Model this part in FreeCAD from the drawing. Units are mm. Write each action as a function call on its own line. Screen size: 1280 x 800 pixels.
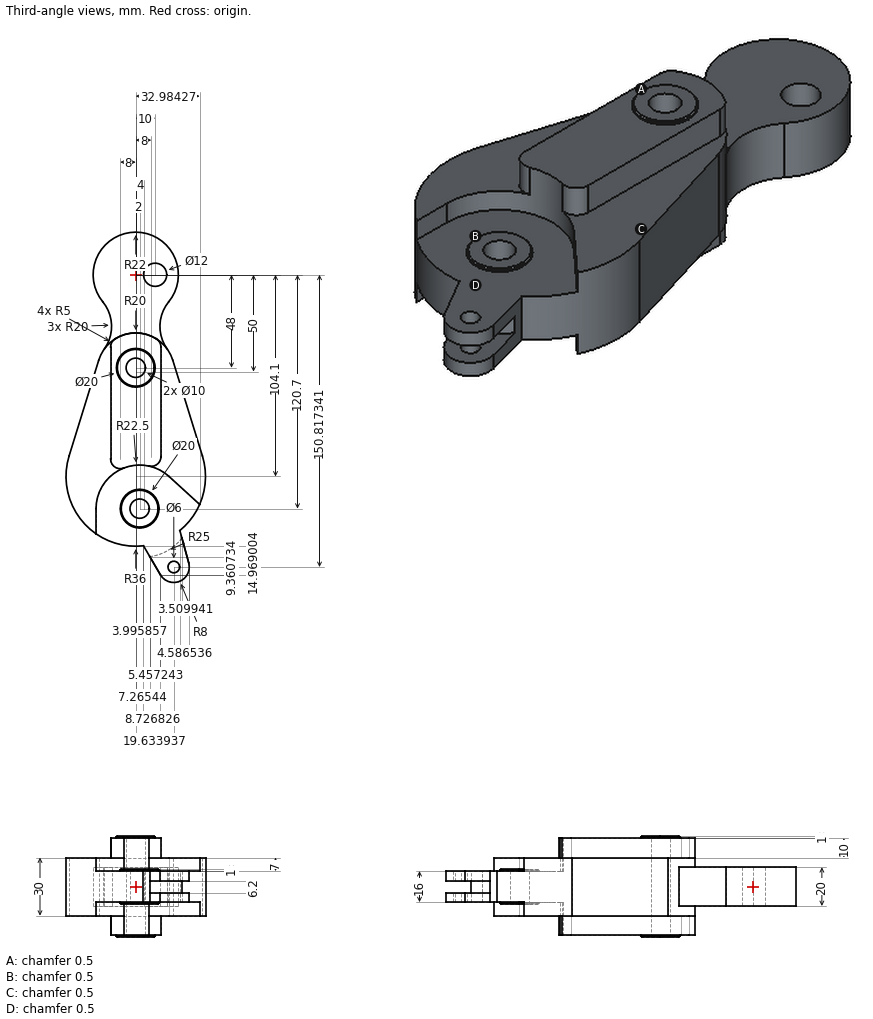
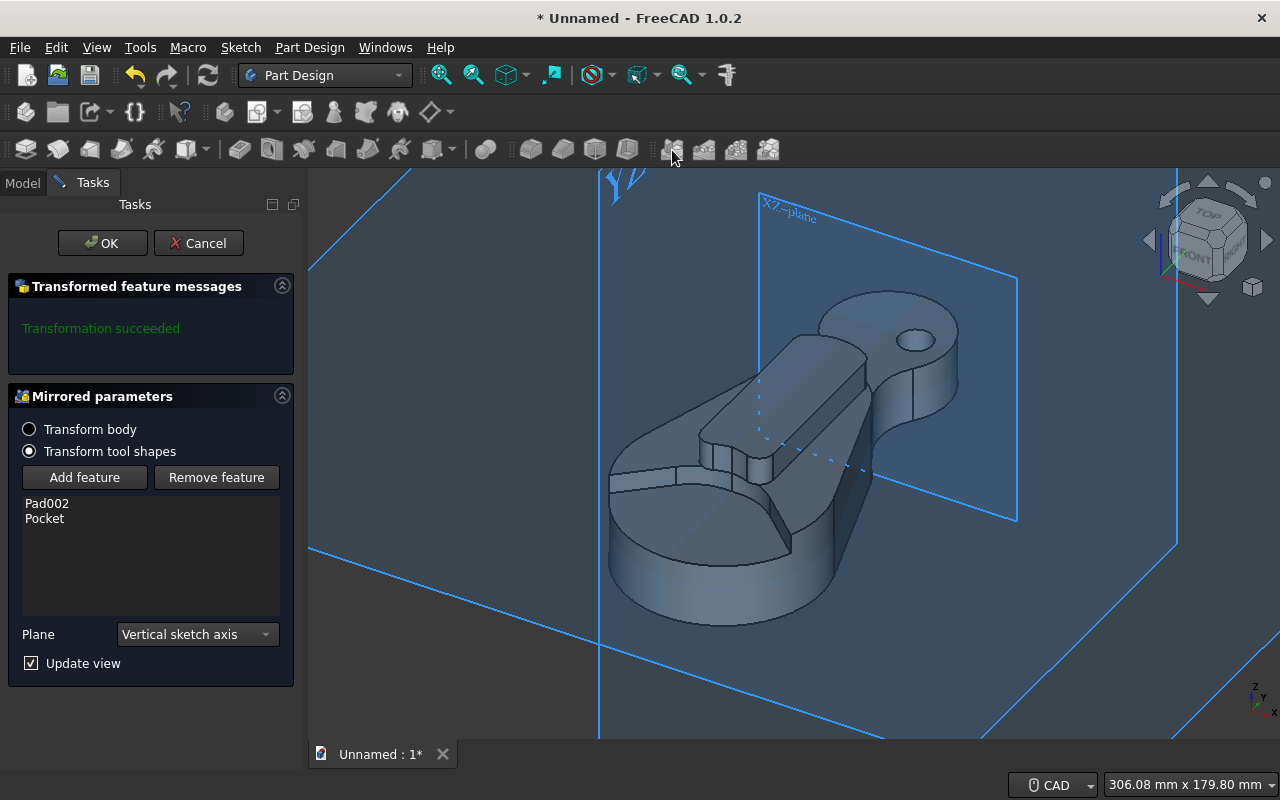
click(198, 634)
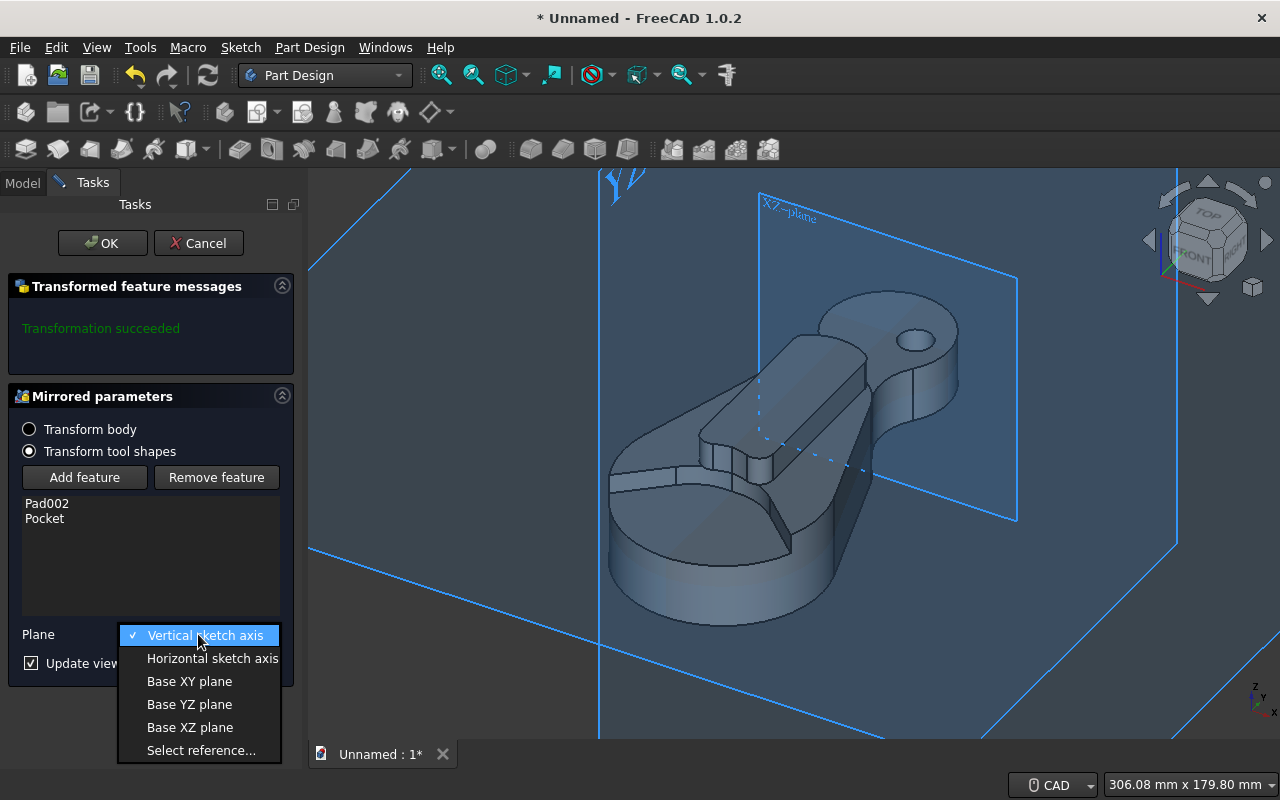
click(198, 682)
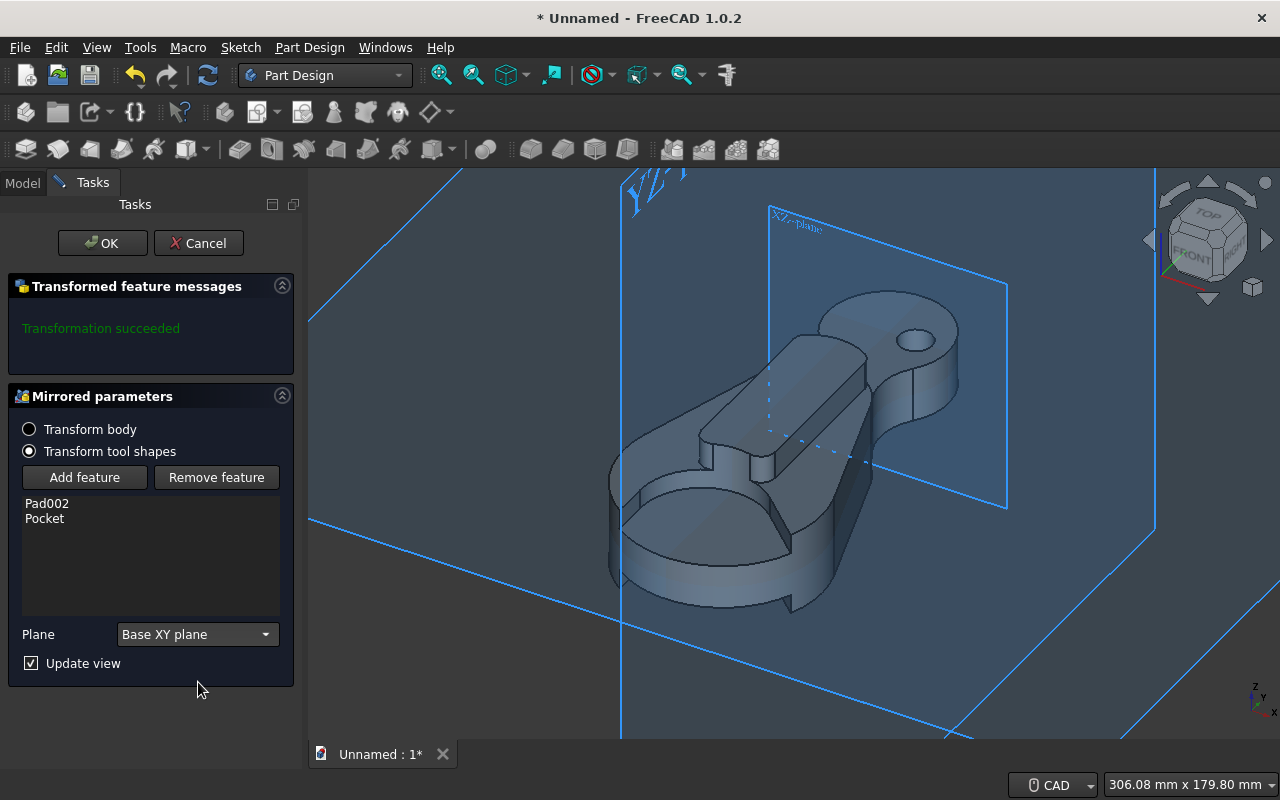
click(103, 243)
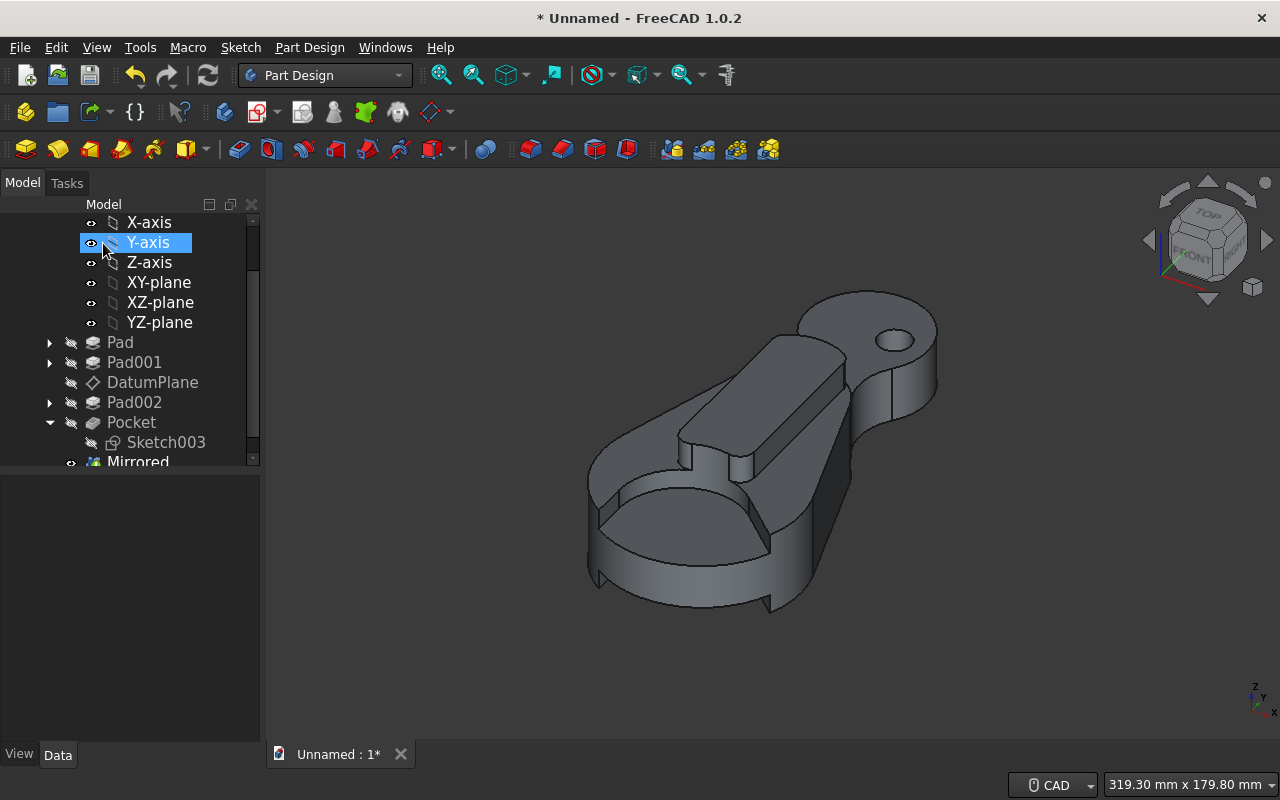
click(796, 362)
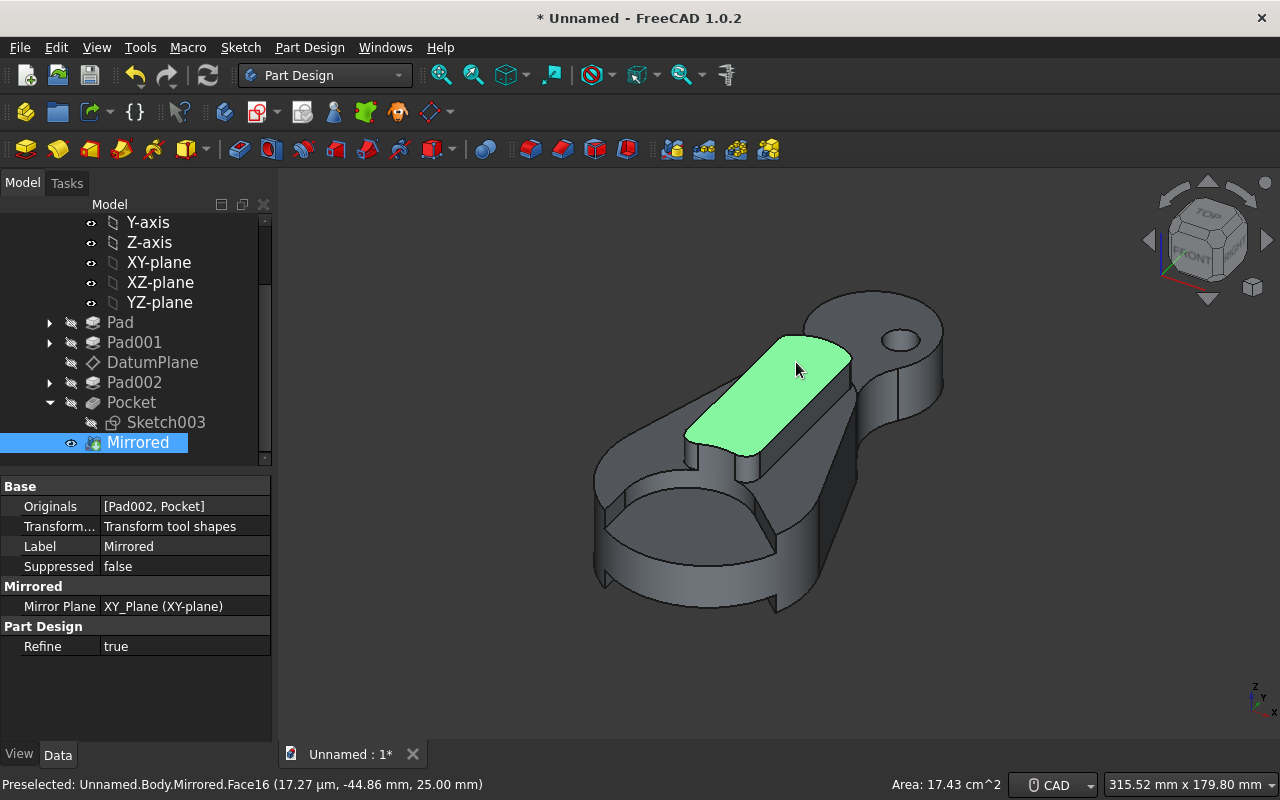
click(258, 112)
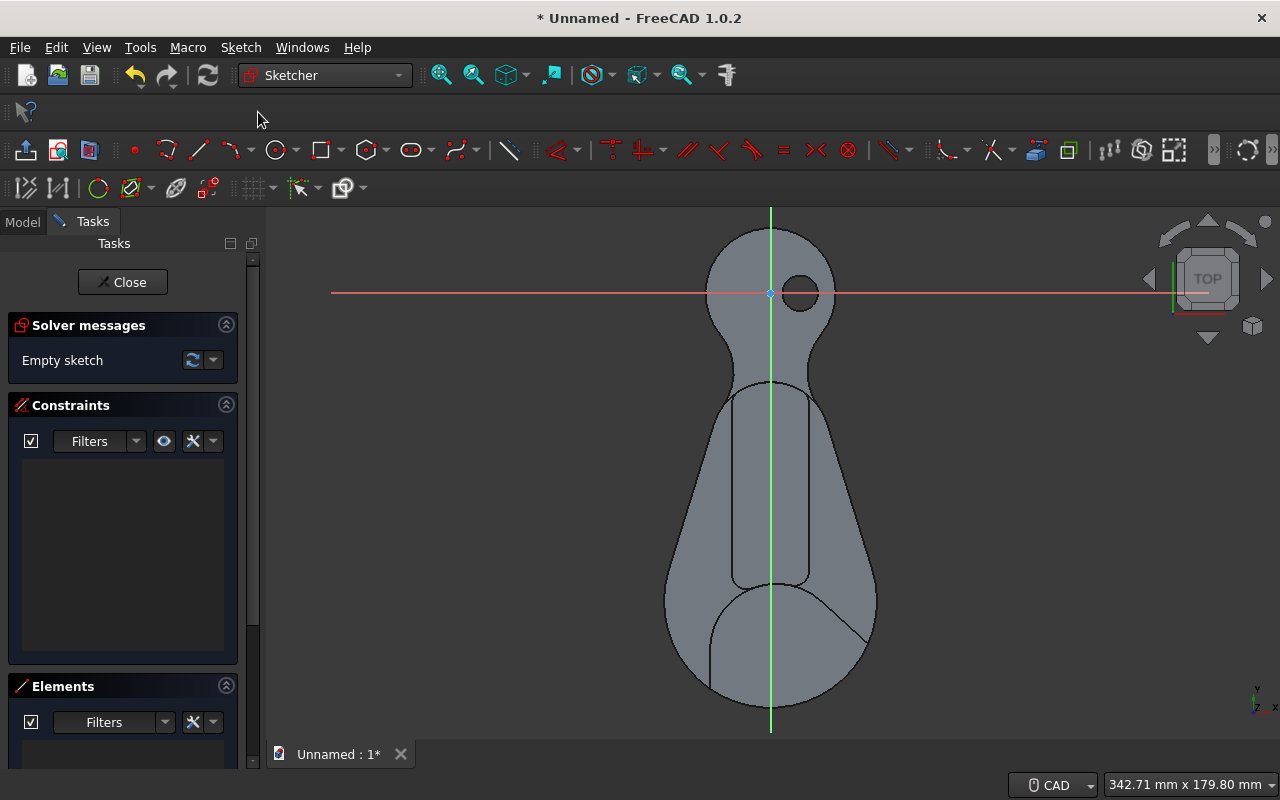
scroll(784, 428, up, 9)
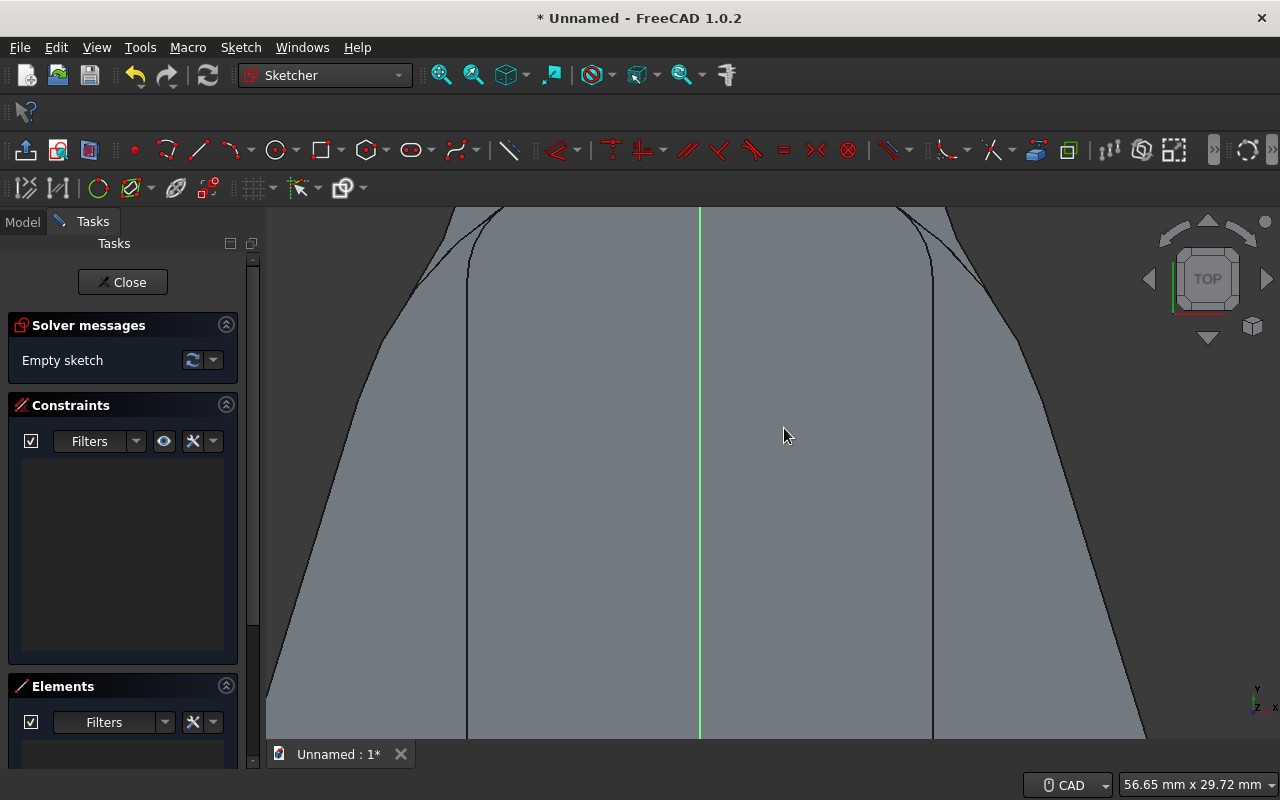
click(276, 150)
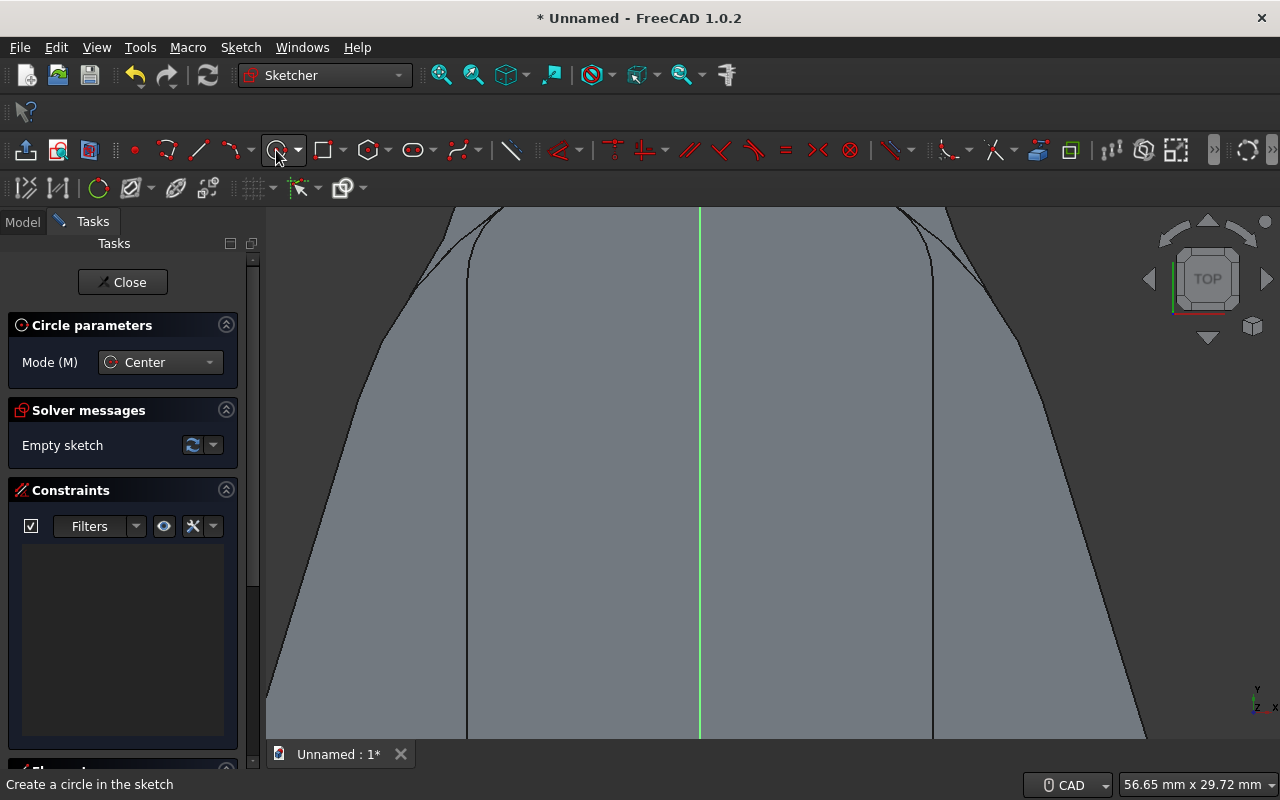
click(700, 470)
click(827, 343)
key(Escape)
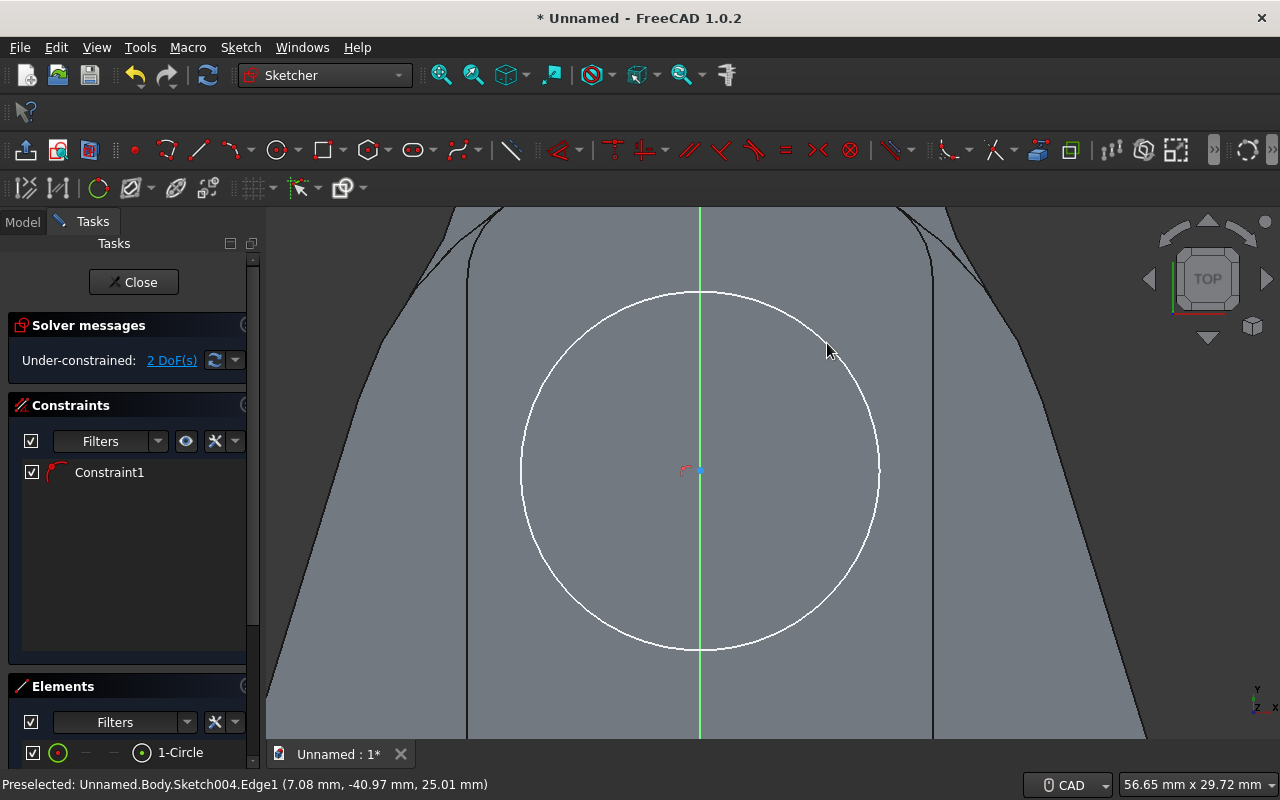
click(558, 150)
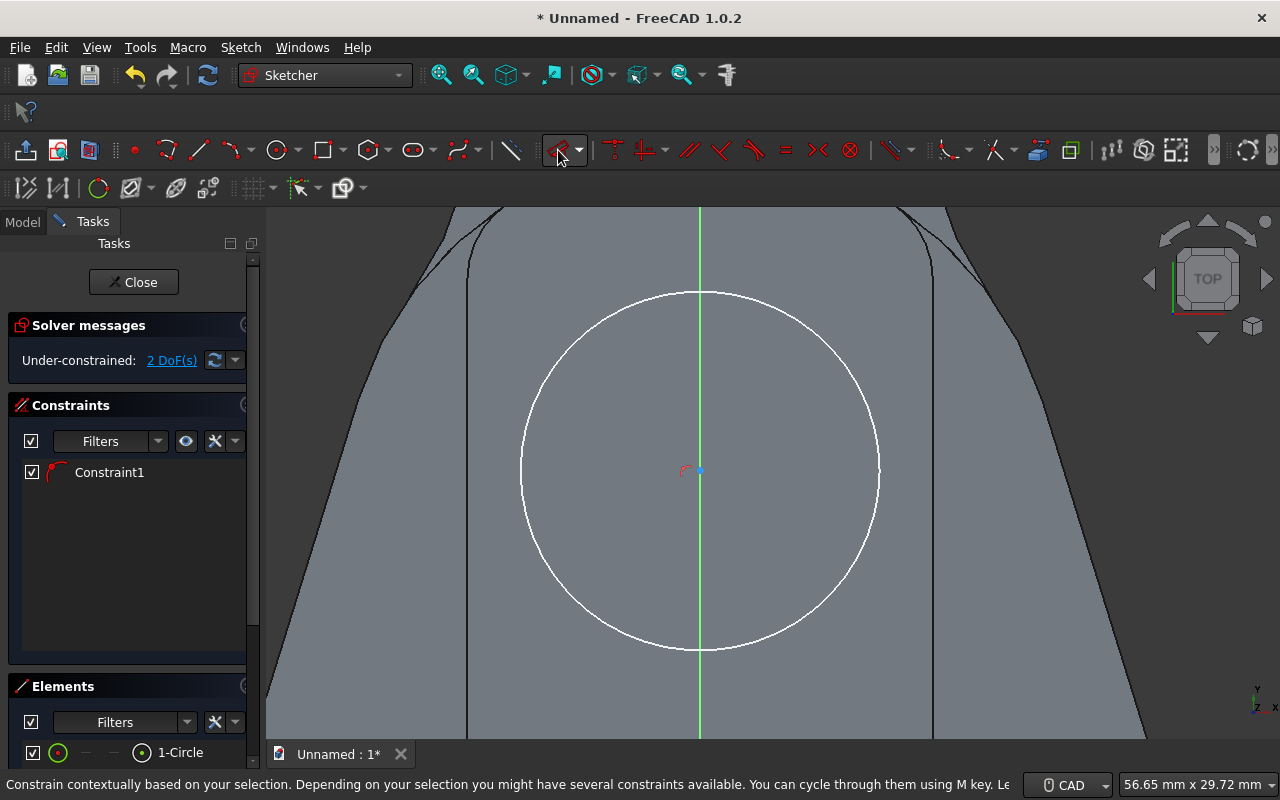
click(827, 344)
click(850, 321)